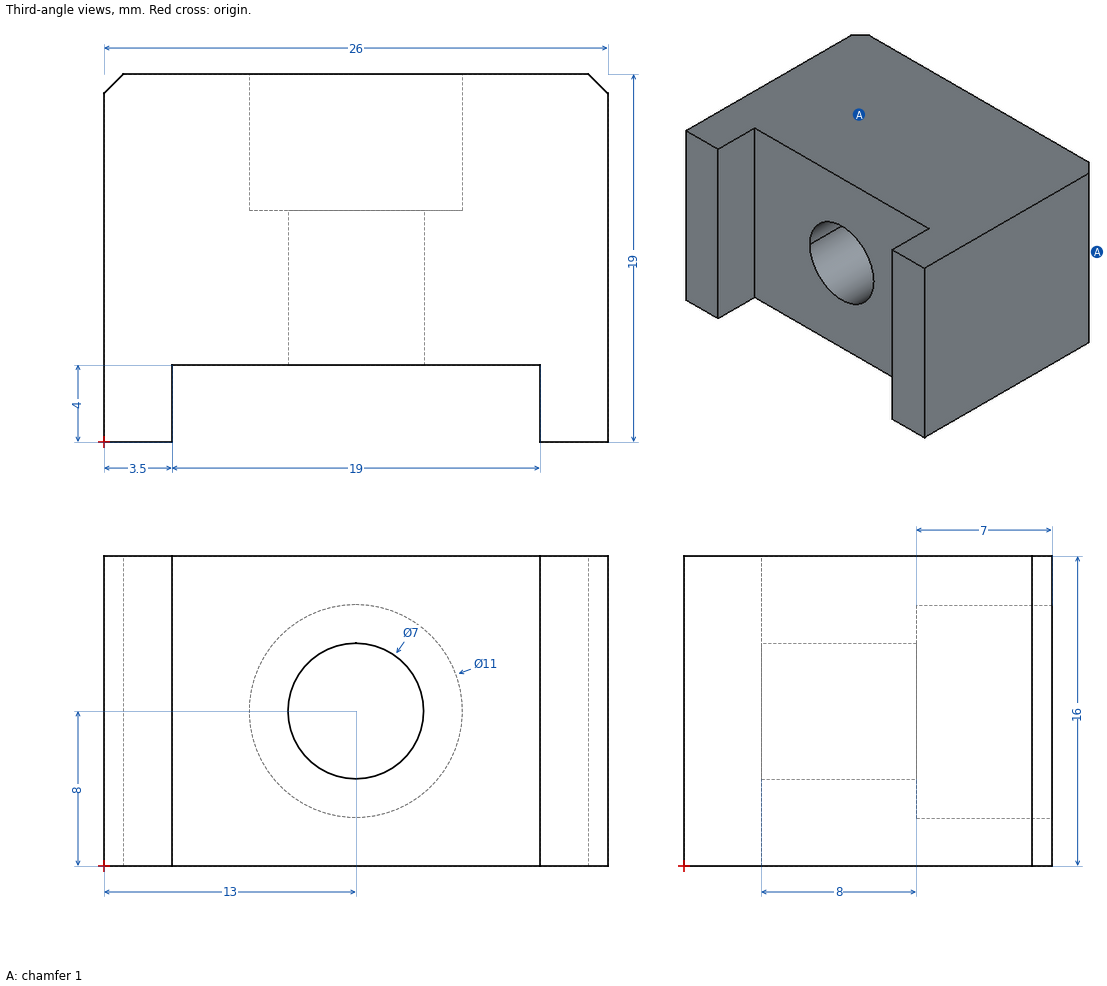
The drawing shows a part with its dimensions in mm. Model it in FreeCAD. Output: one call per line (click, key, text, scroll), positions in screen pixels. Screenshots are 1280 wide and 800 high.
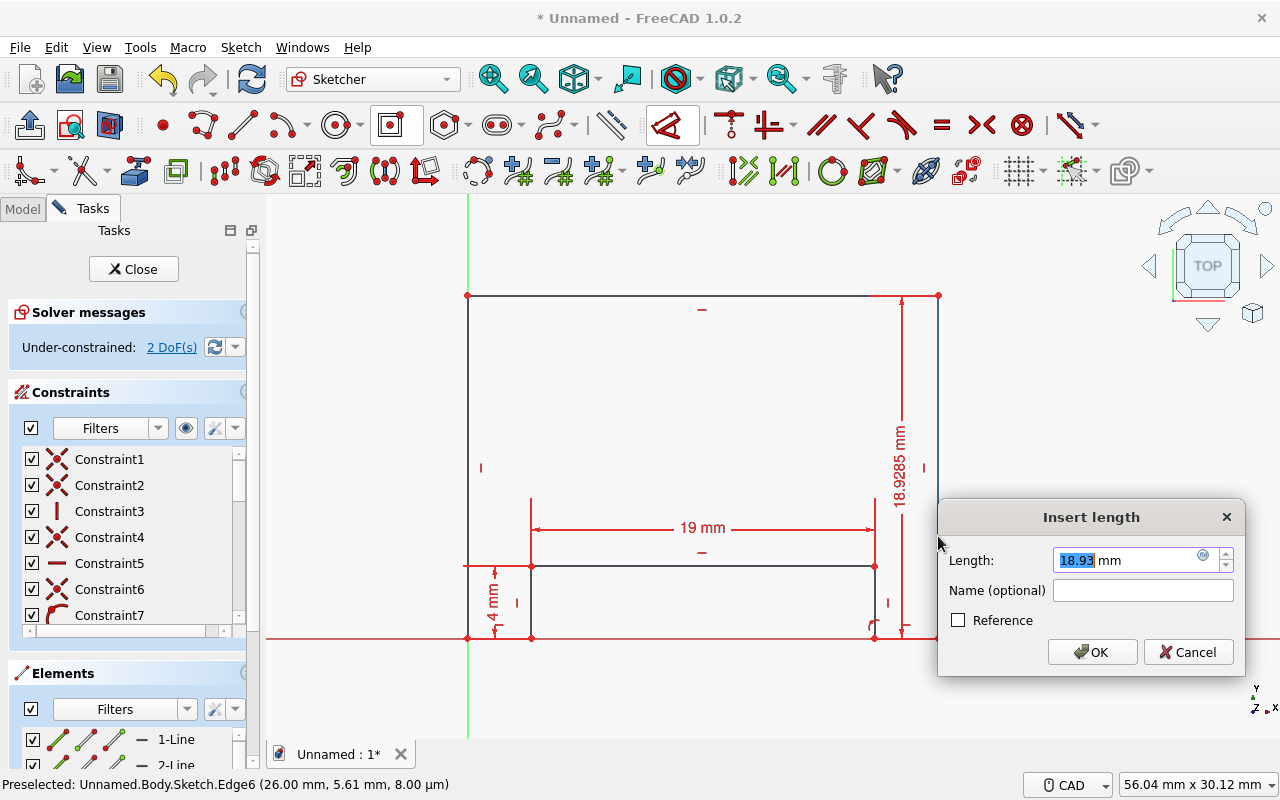
text(19)
key(Return)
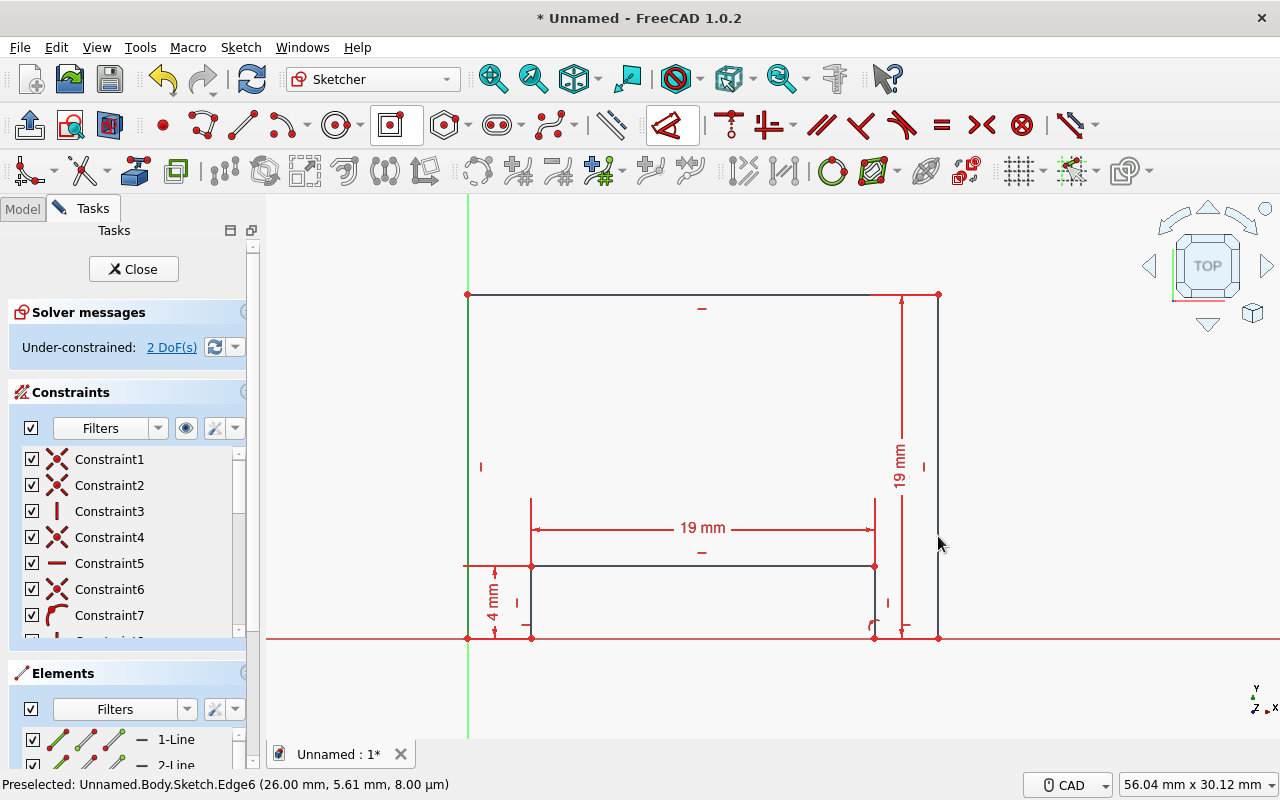
click(797, 295)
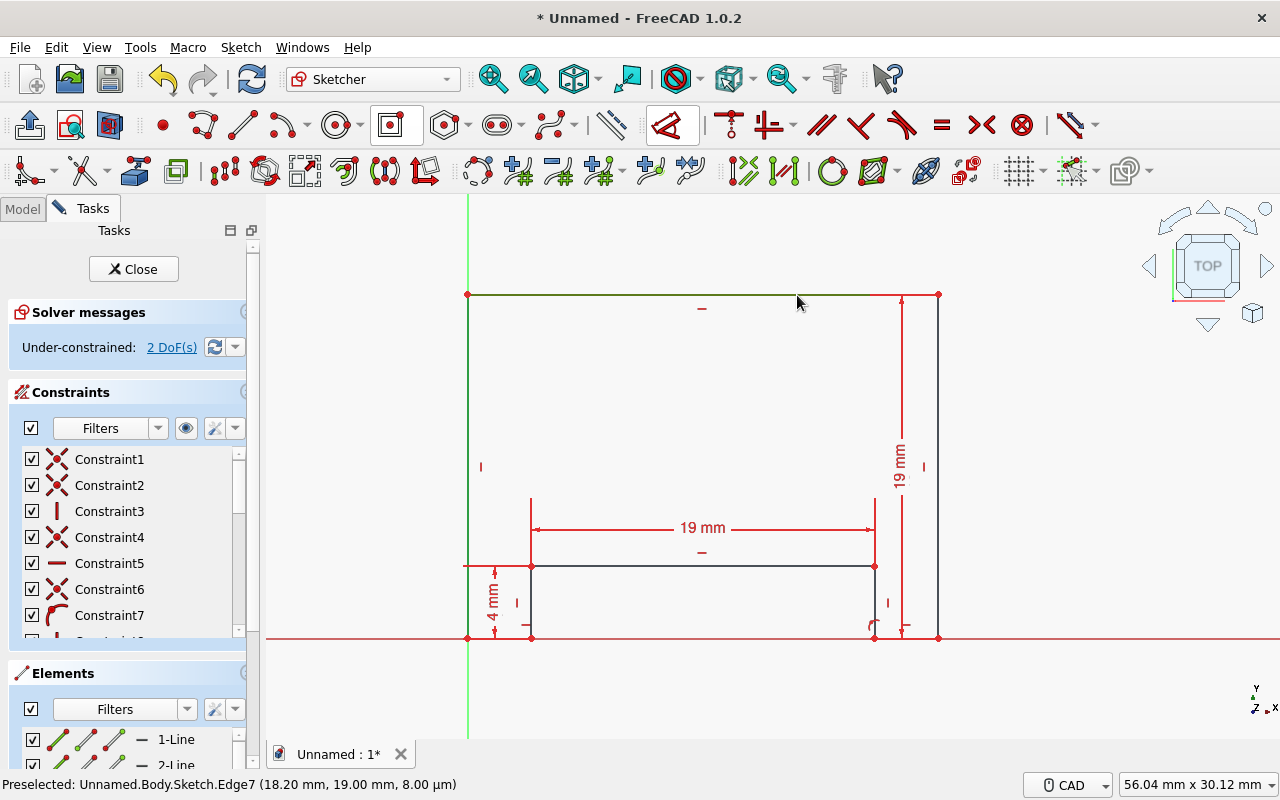
key(l)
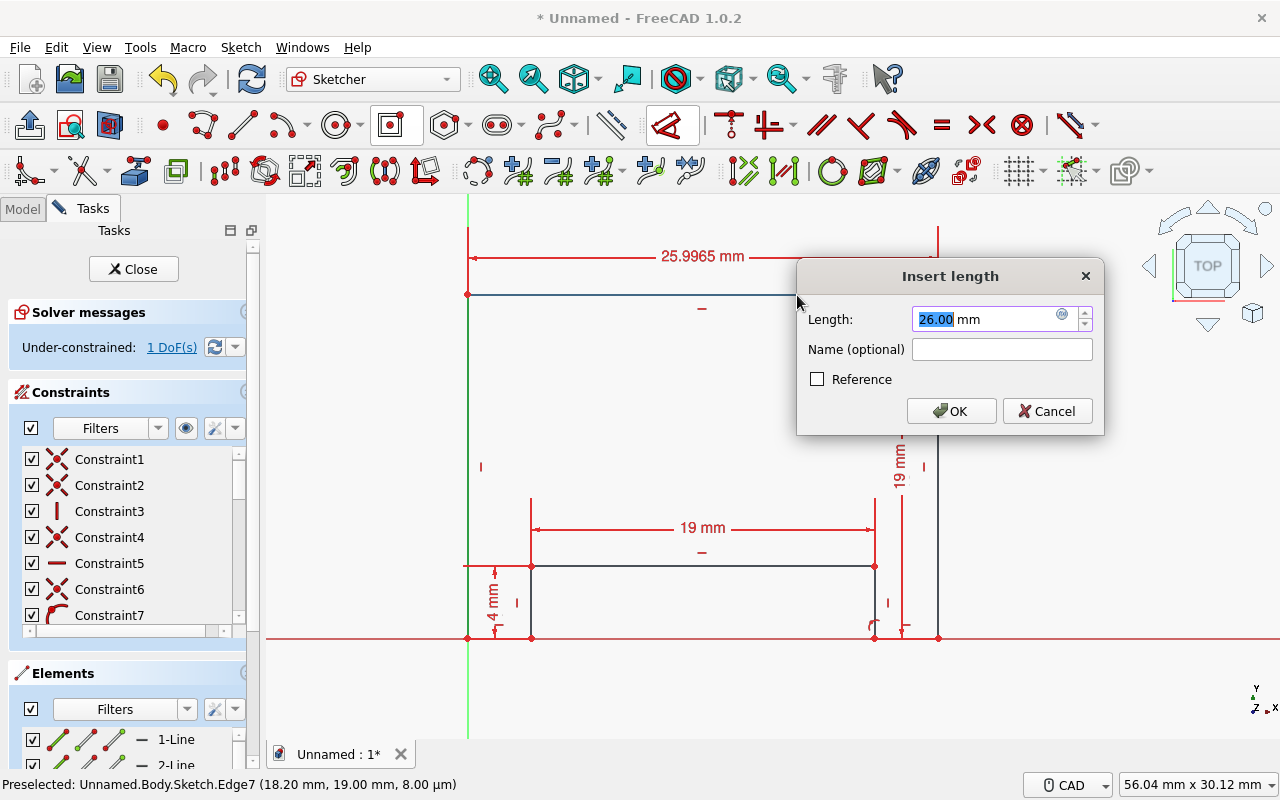
text(26)
key(Return)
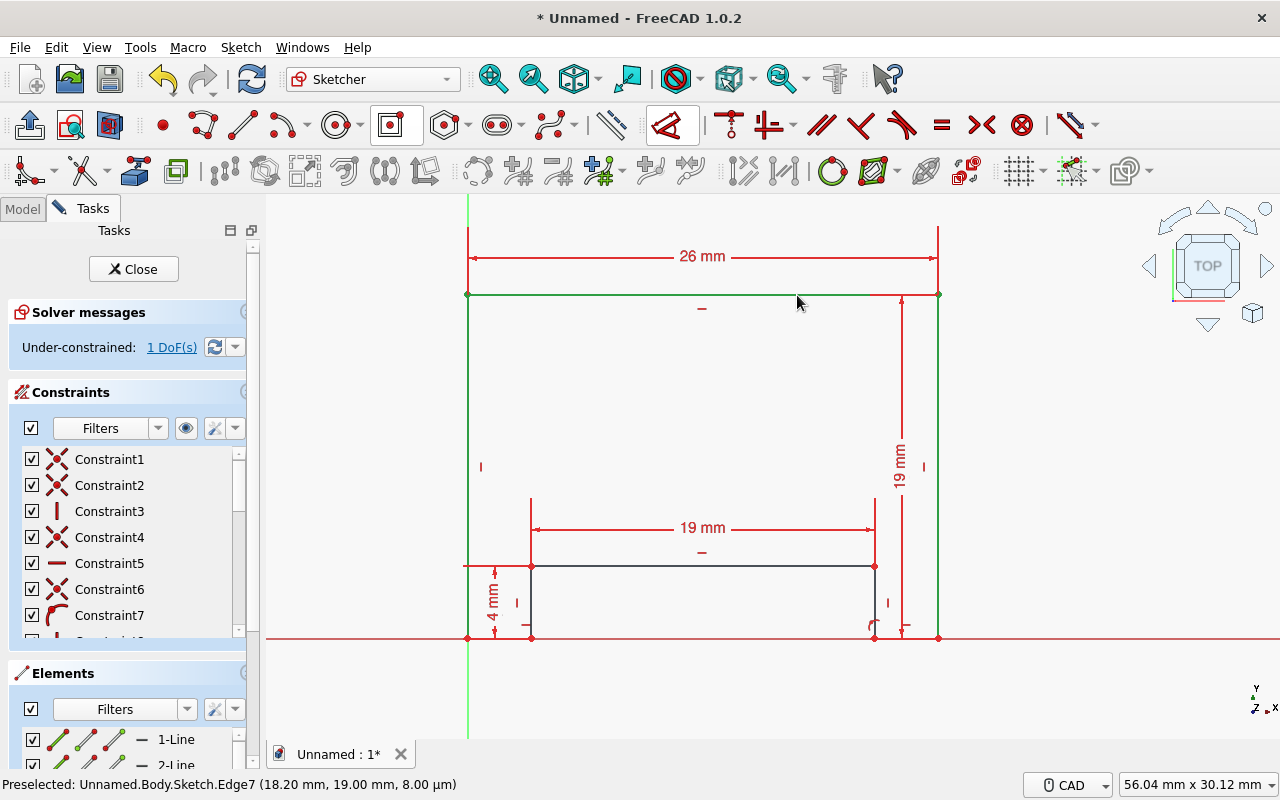
click(487, 639)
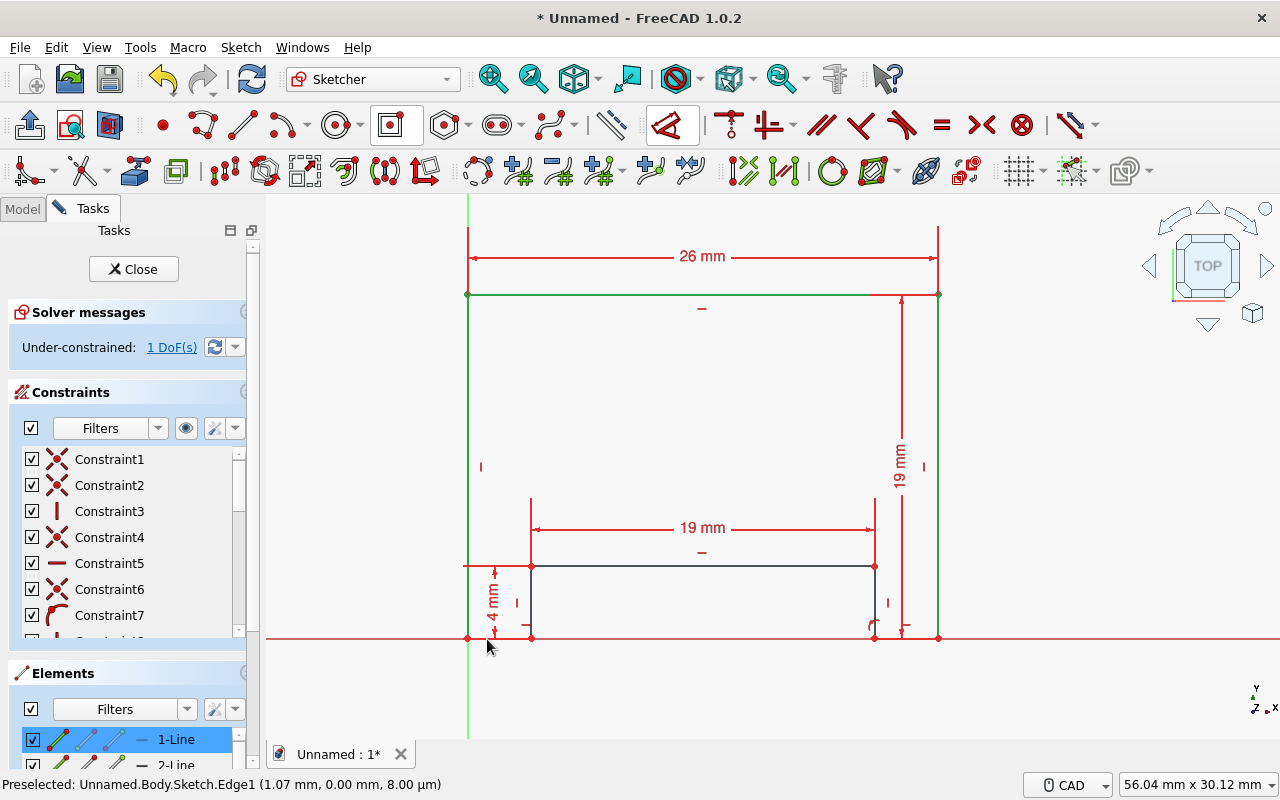
click(694, 126)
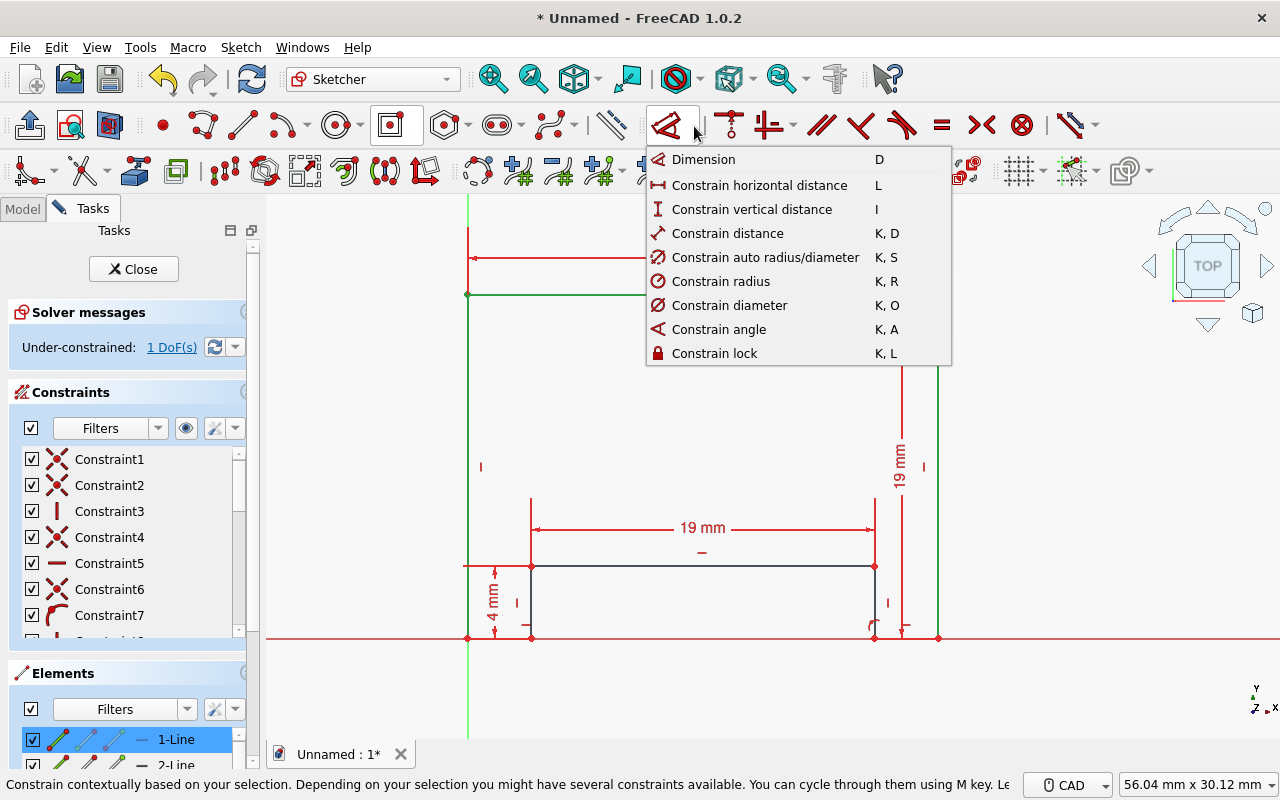
click(799, 185)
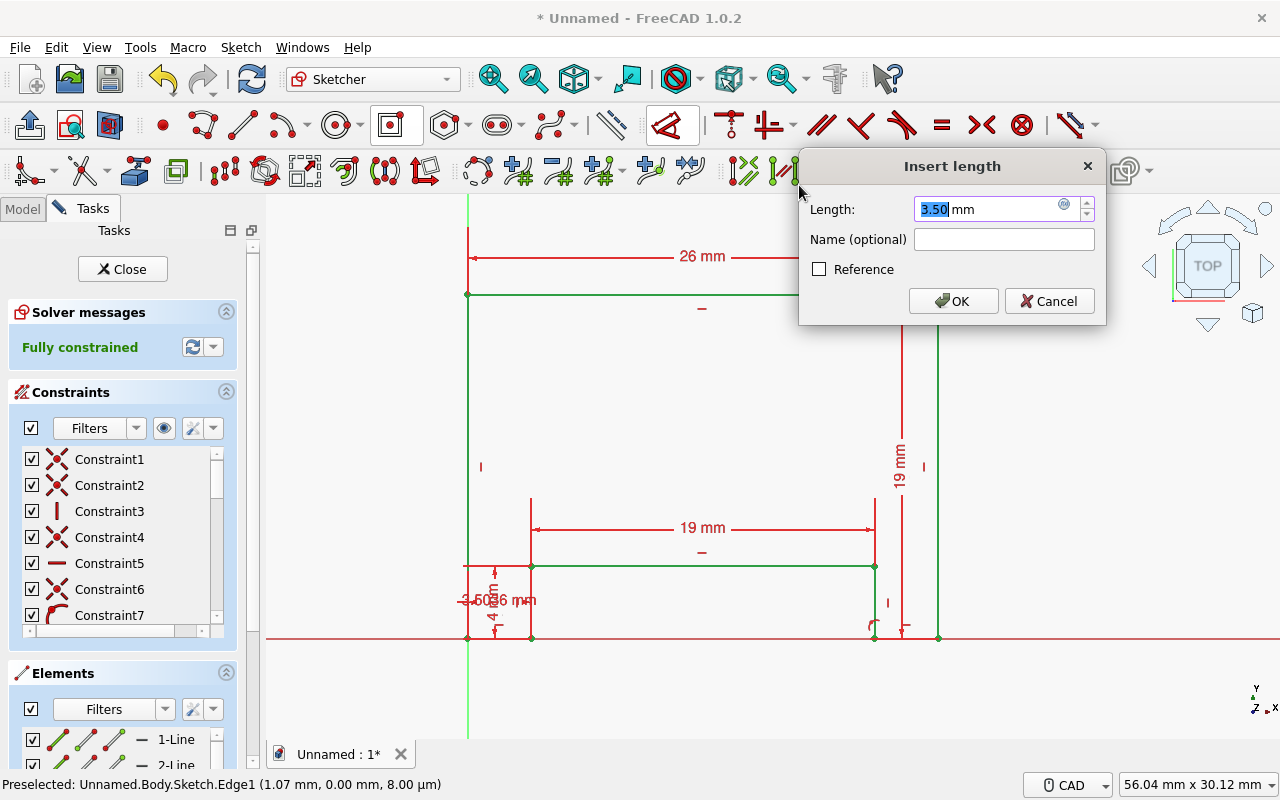
text(3.5)
key(Return)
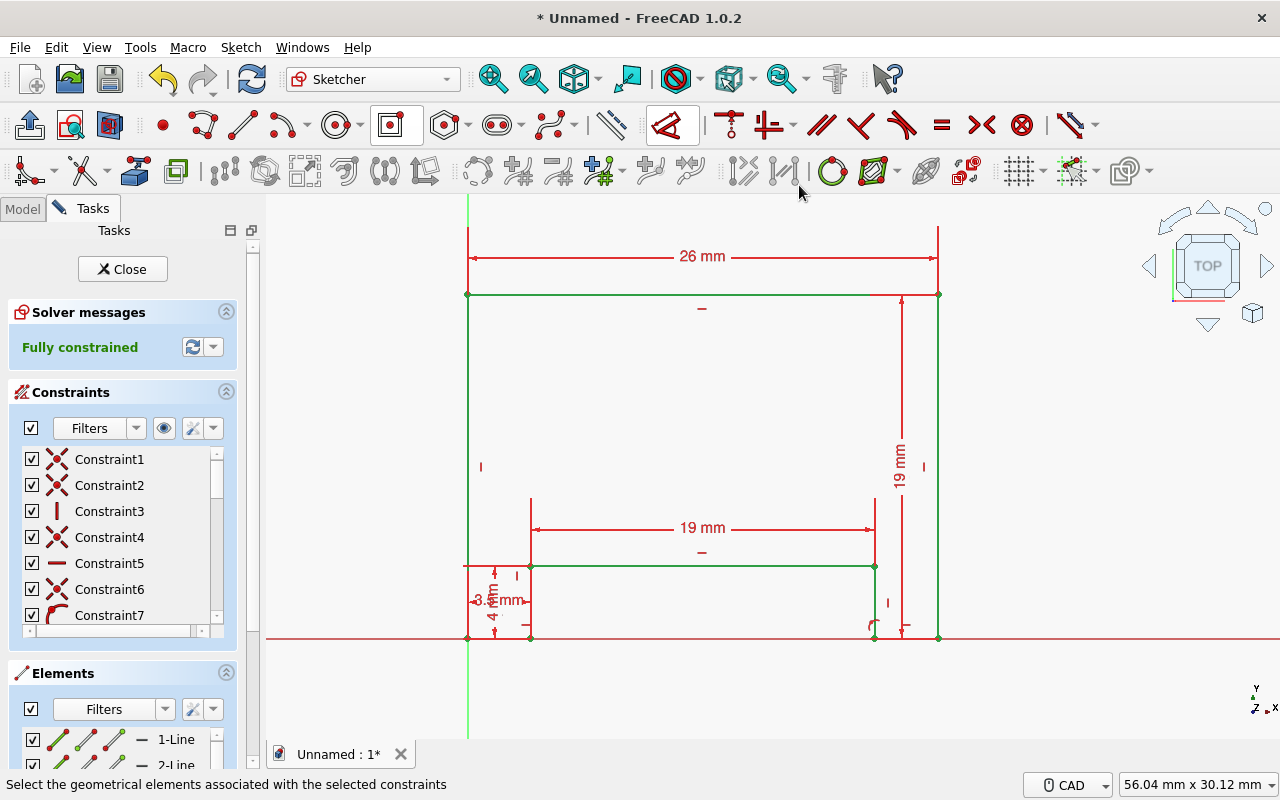
click(123, 269)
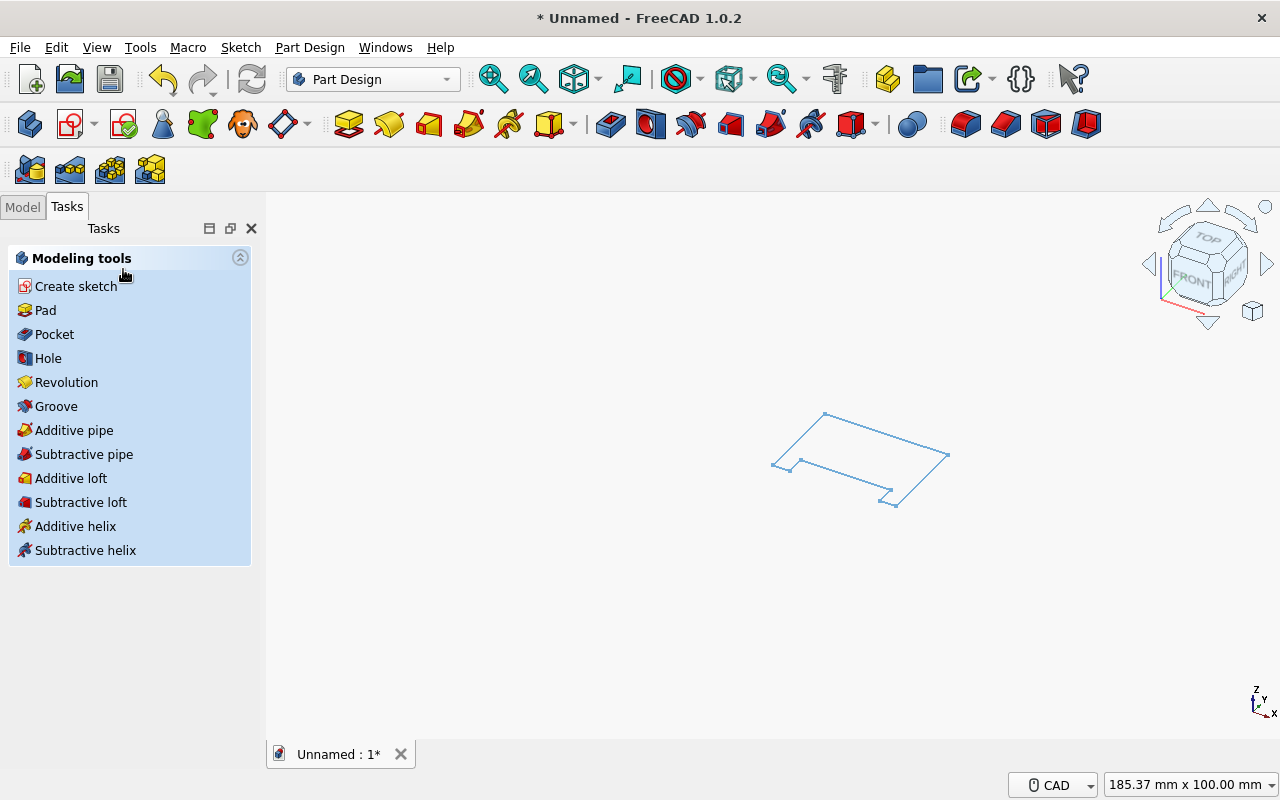
click(350, 124)